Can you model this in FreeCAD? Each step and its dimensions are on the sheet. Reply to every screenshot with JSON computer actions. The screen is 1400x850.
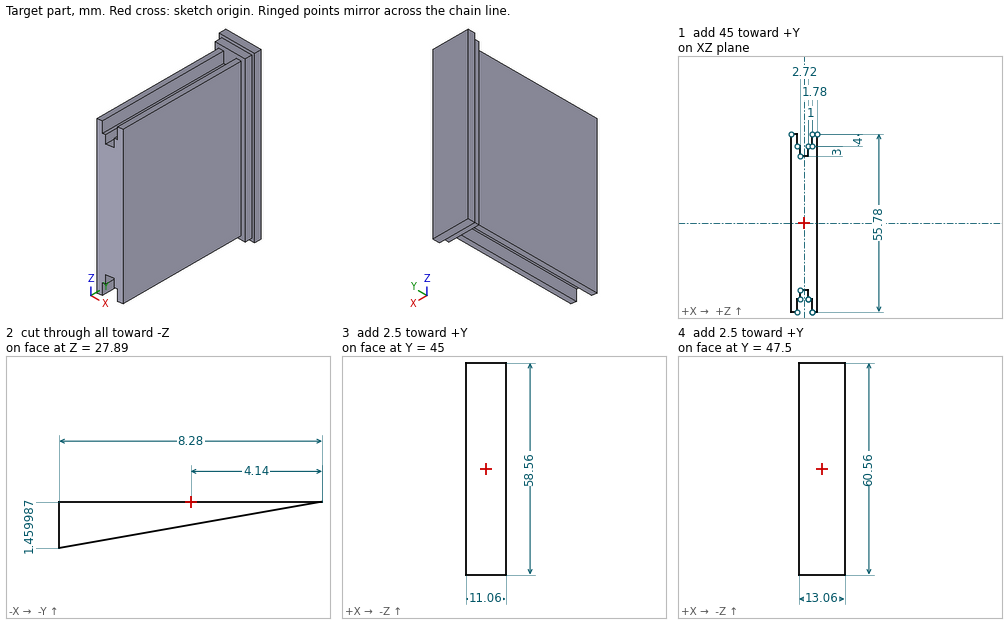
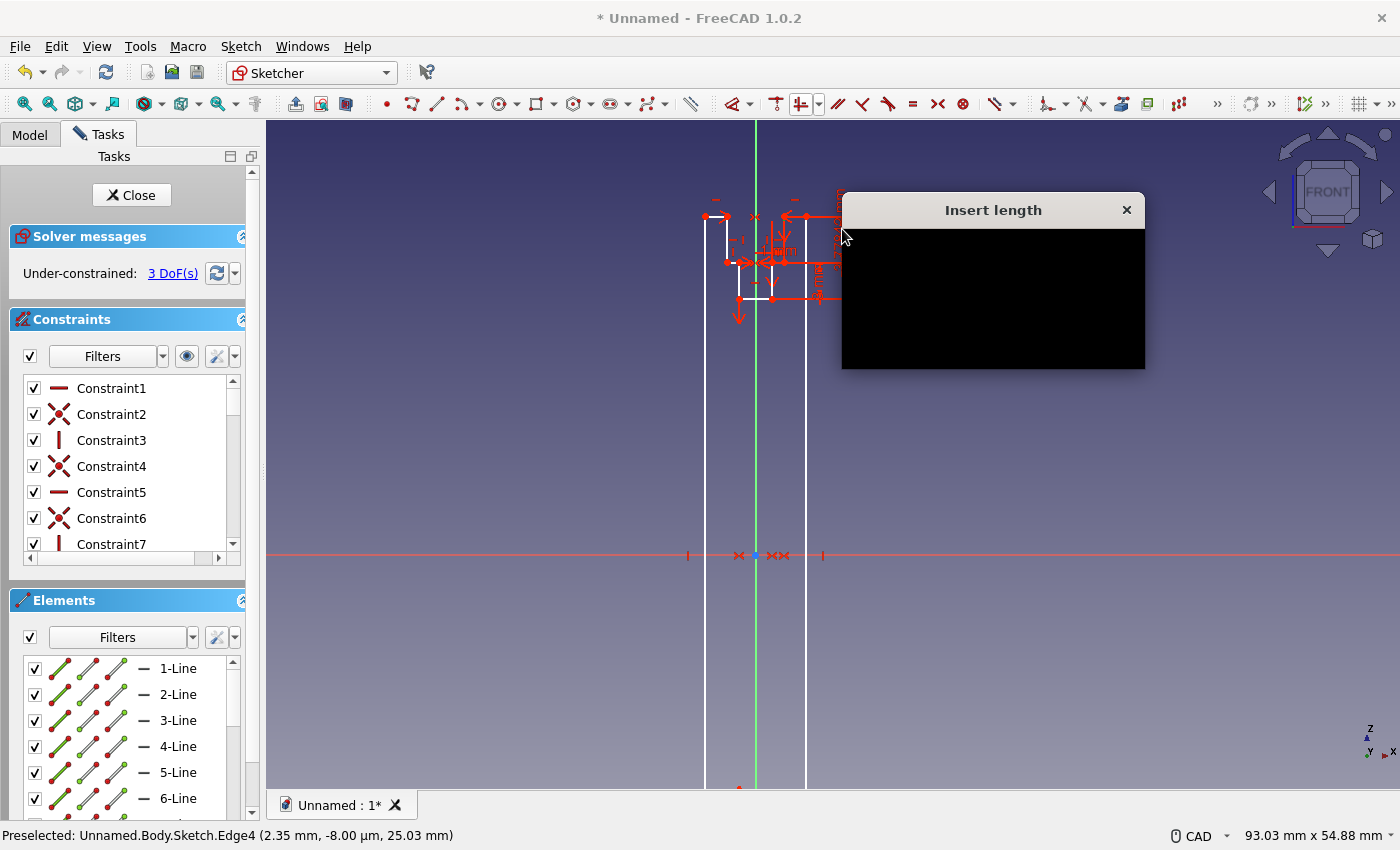
{"action": "type", "text": "4"}
{"action": "key", "text": "Return"}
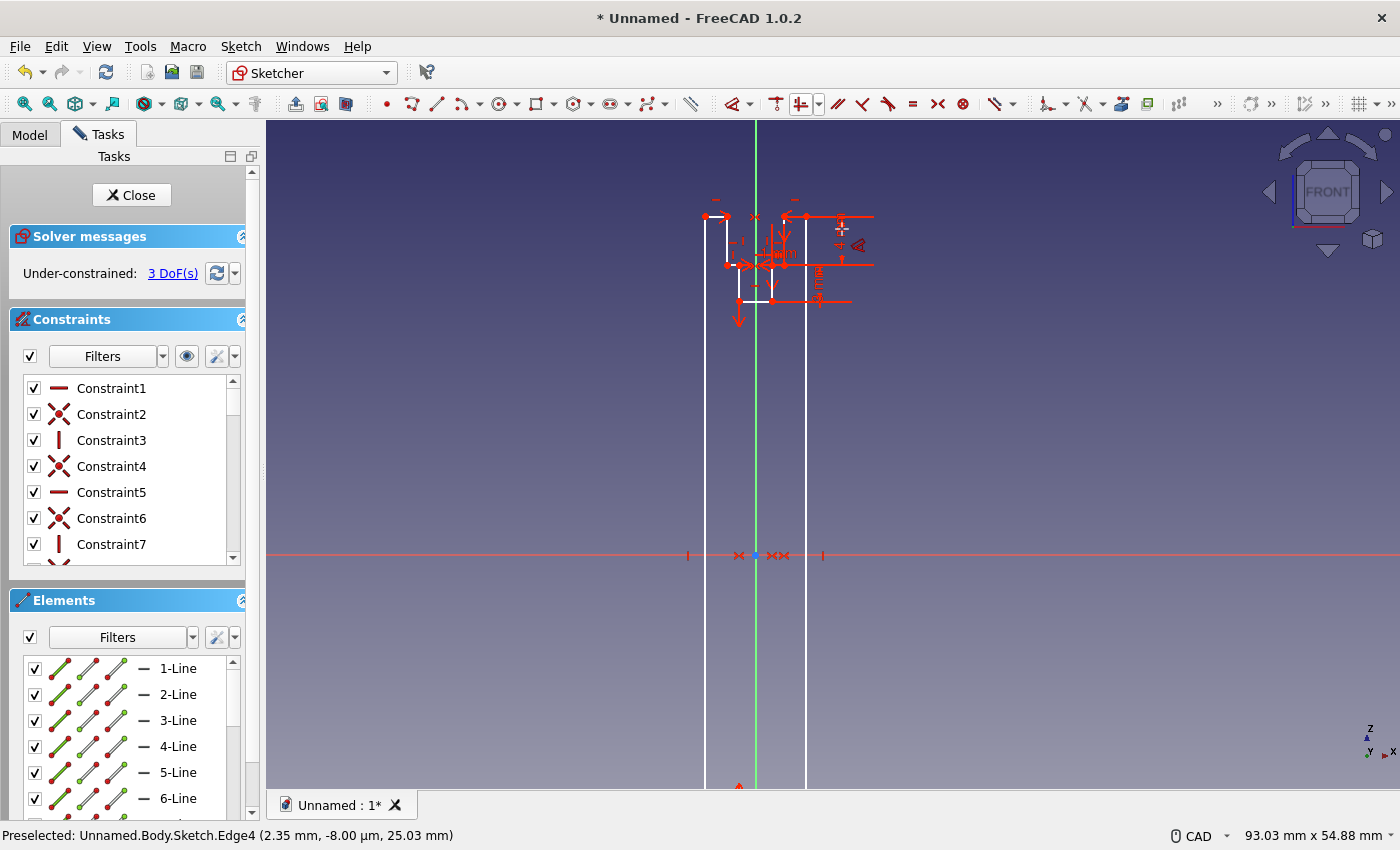
{"action": "left_click", "coordinate": [752, 302]}
{"action": "left_click", "coordinate": [748, 268]}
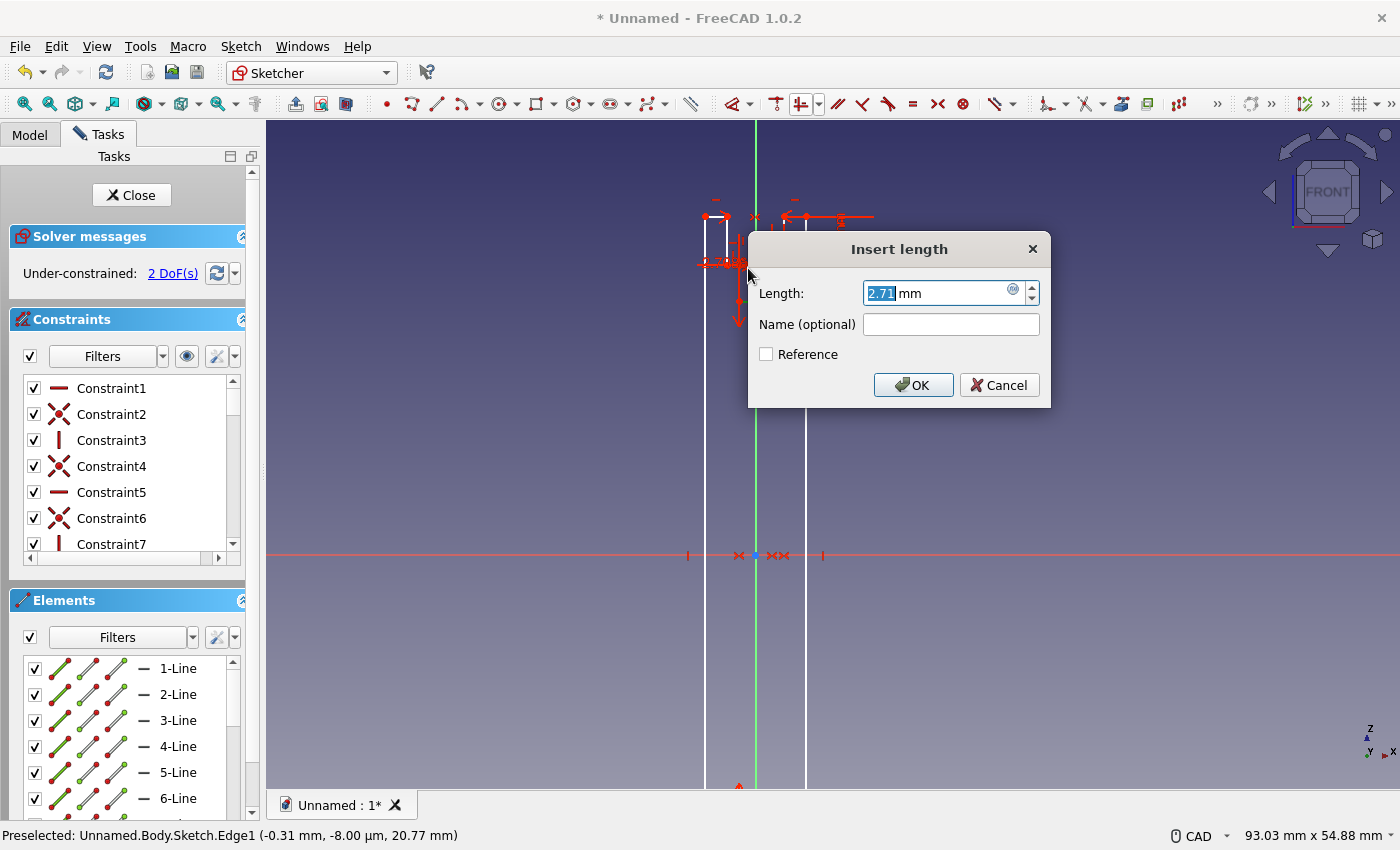
{"action": "type", "text": "2.72"}
{"action": "key", "text": "Return"}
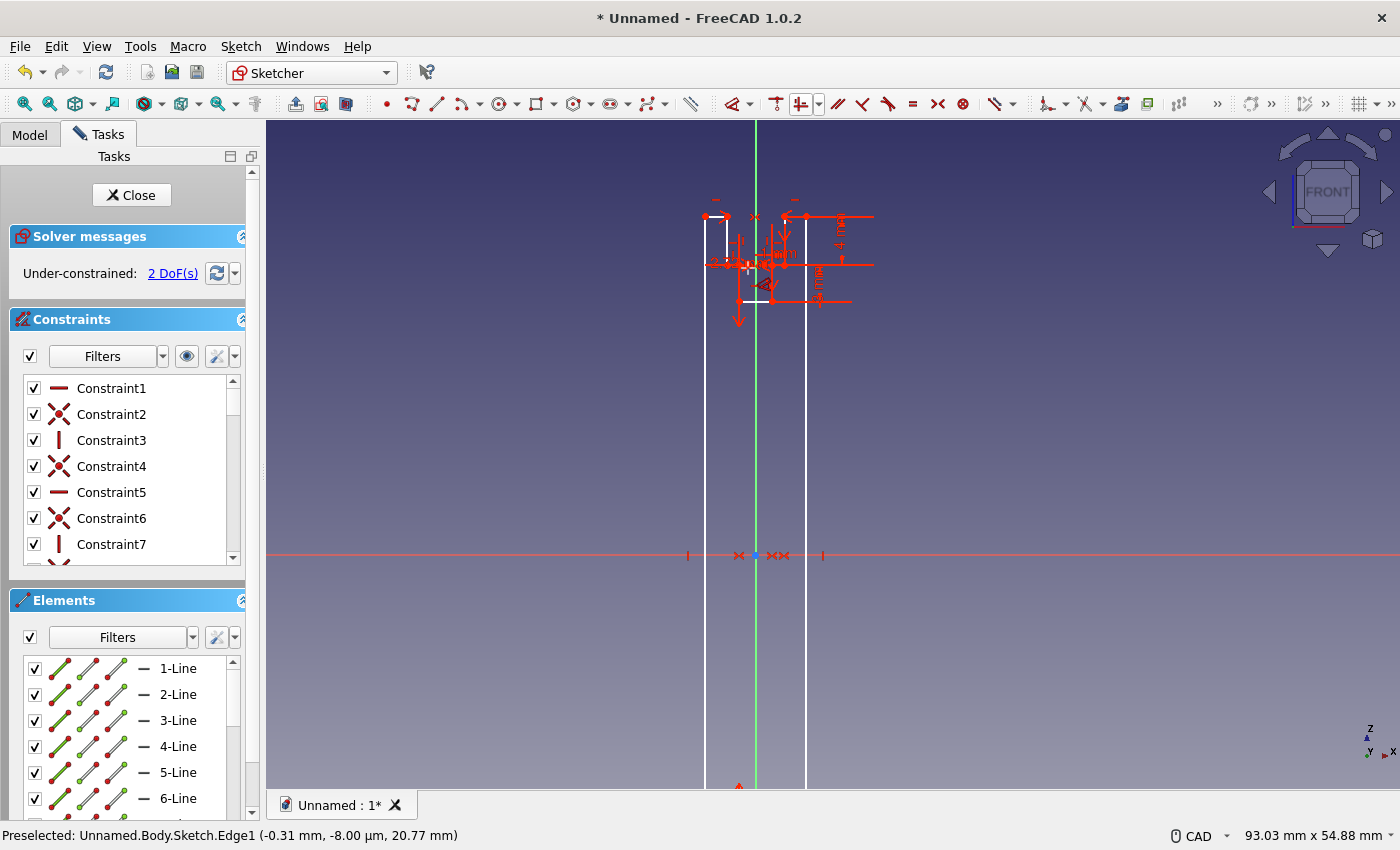
{"action": "scroll", "coordinate": [795, 217], "scroll_direction": "up", "scroll_amount": 4}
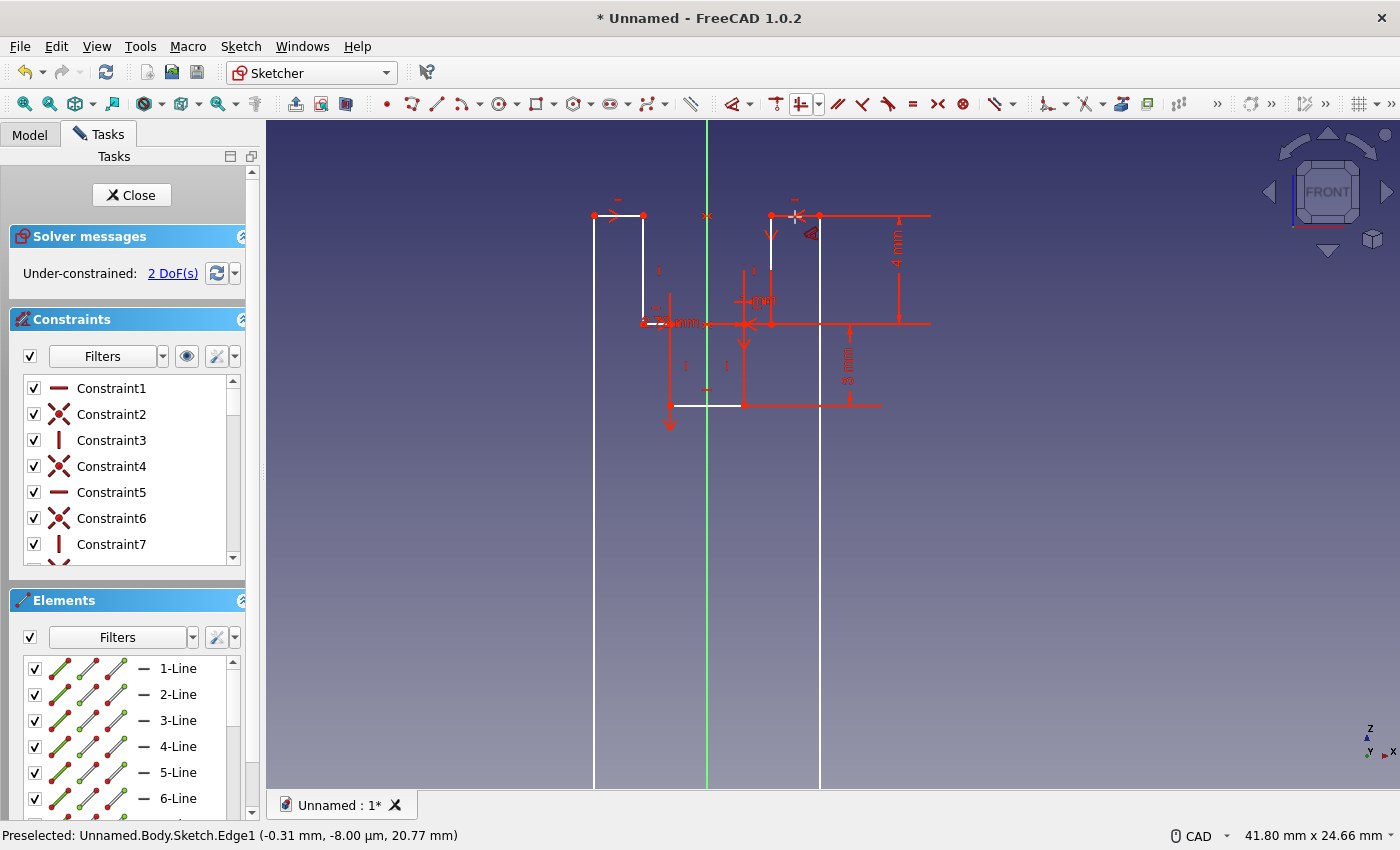
{"action": "left_click", "coordinate": [796, 216]}
{"action": "left_click", "coordinate": [796, 182]}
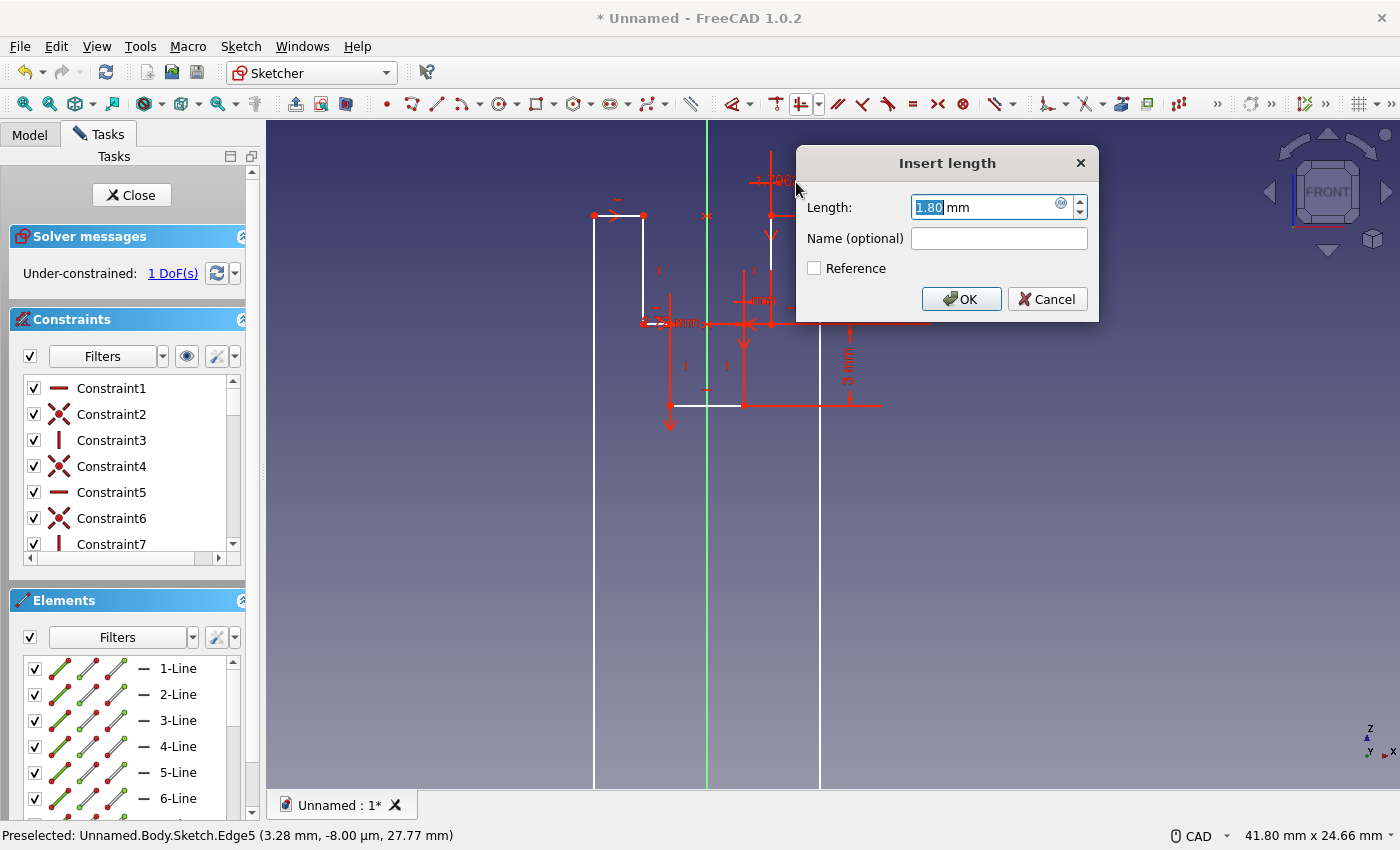
{"action": "type", "text": "1.78"}
{"action": "key", "text": "Return"}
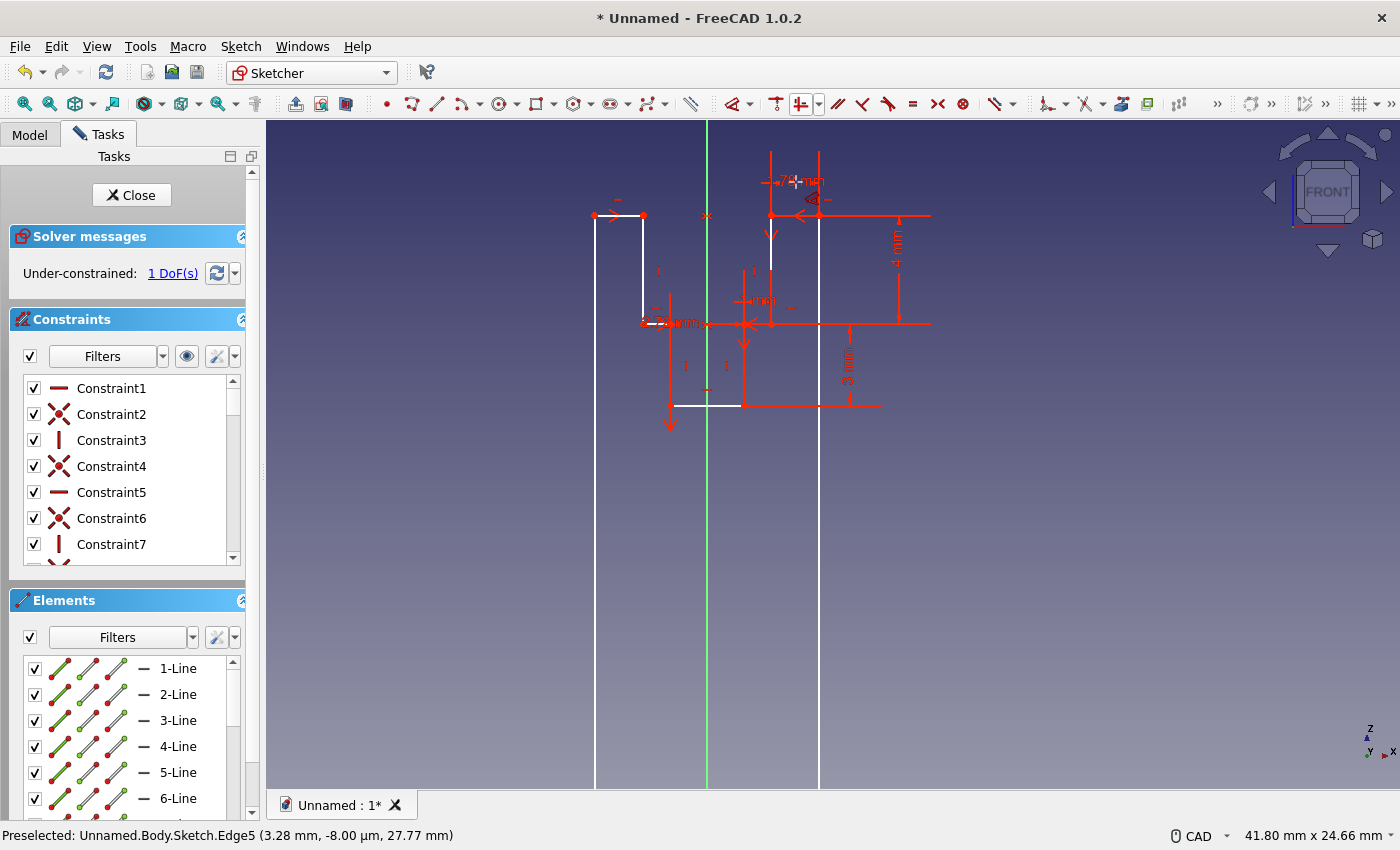
{"action": "scroll", "coordinate": [789, 233], "scroll_direction": "down", "scroll_amount": 6}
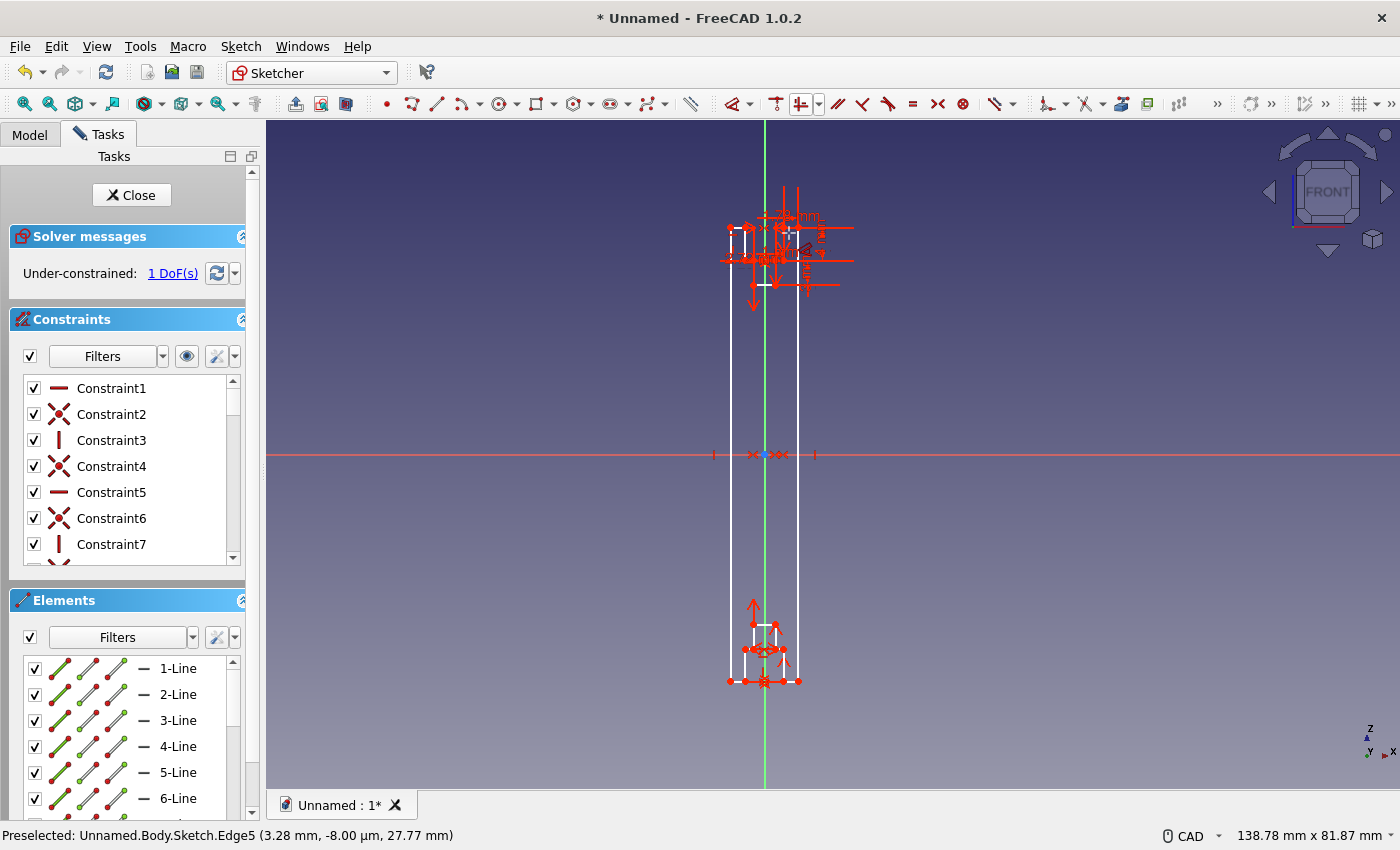
{"action": "left_click", "coordinate": [798, 364]}
{"action": "left_click", "coordinate": [832, 351]}